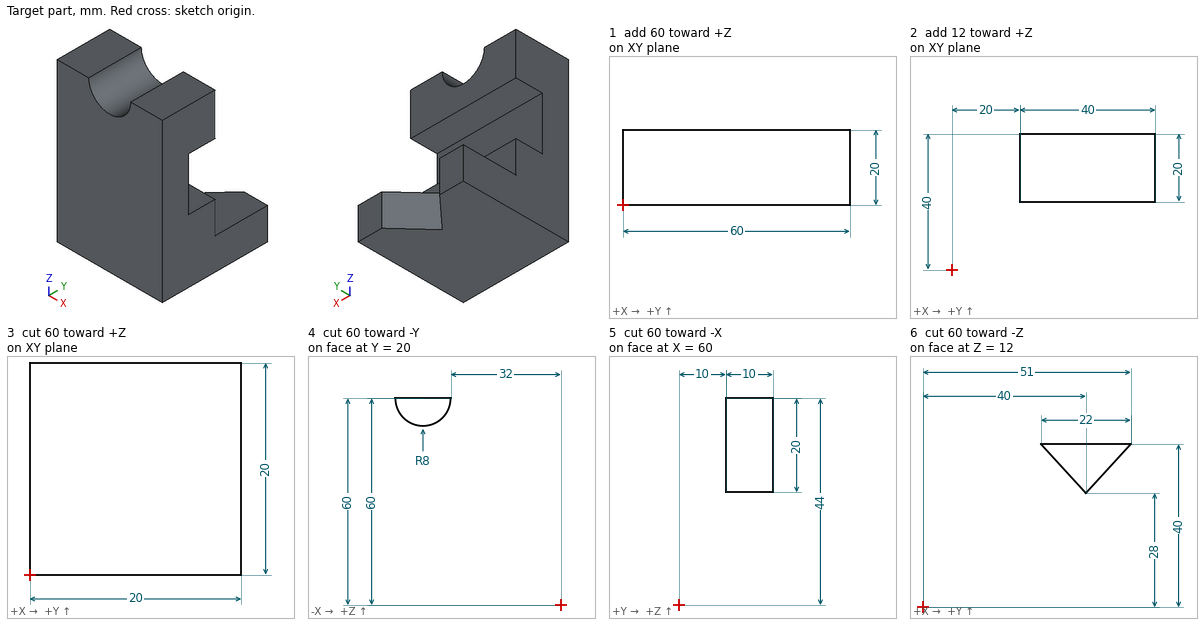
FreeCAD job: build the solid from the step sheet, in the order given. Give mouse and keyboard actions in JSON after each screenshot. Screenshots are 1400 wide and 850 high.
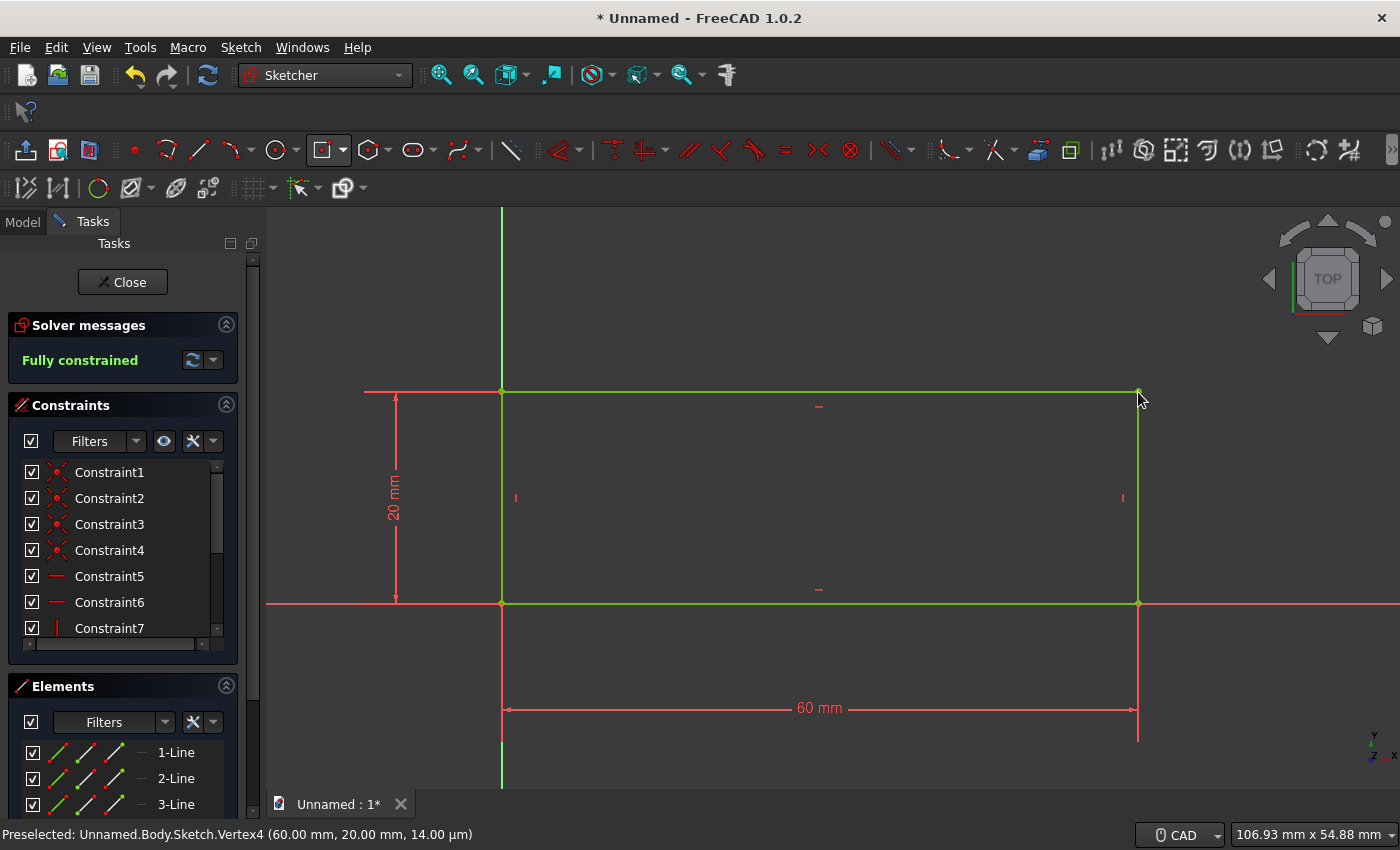
{"action": "left_click", "coordinate": [123, 282]}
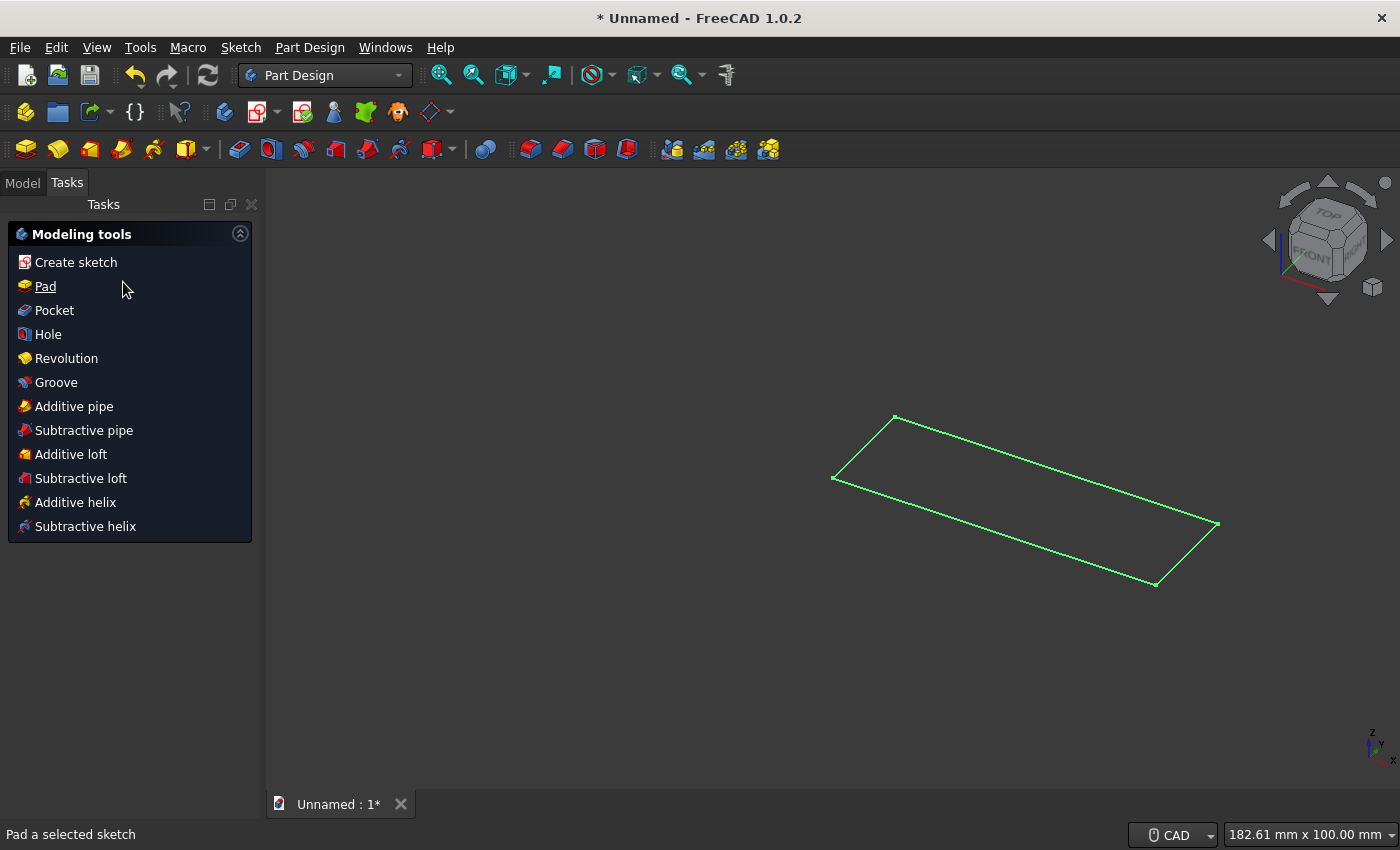
{"action": "left_click", "coordinate": [26, 150]}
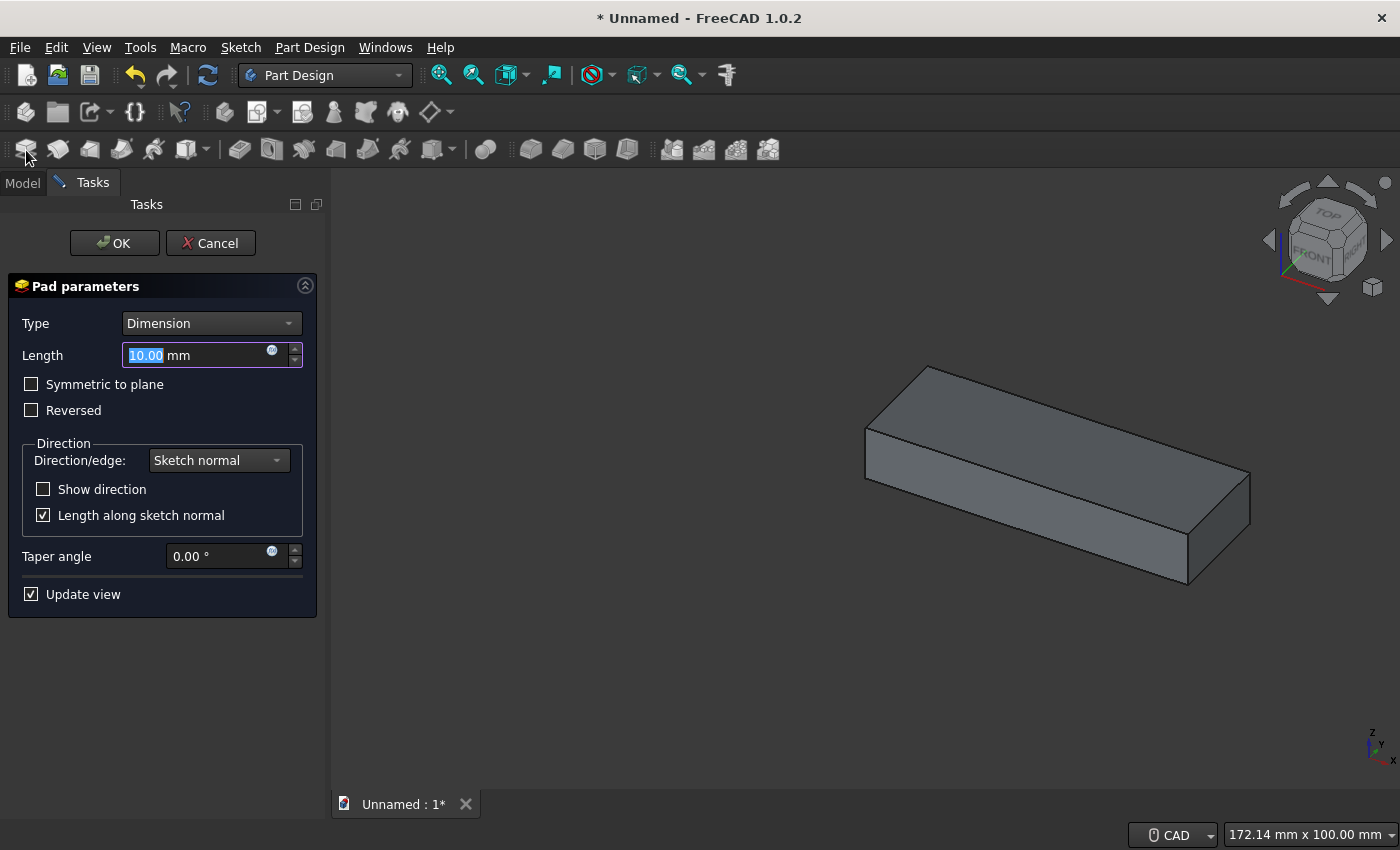
{"action": "type", "text": "60"}
{"action": "key", "text": "Tab"}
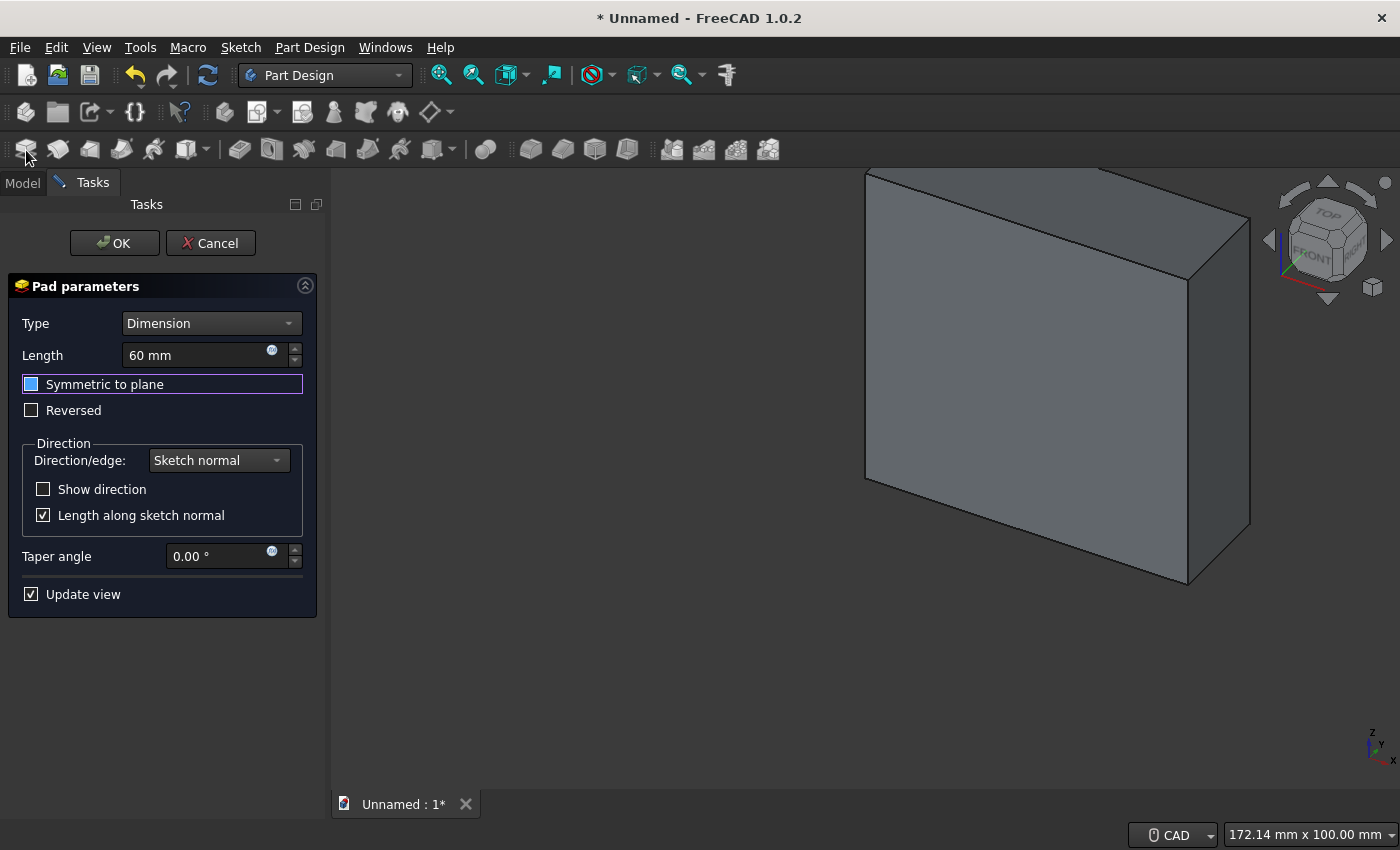
{"action": "left_click", "coordinate": [115, 243]}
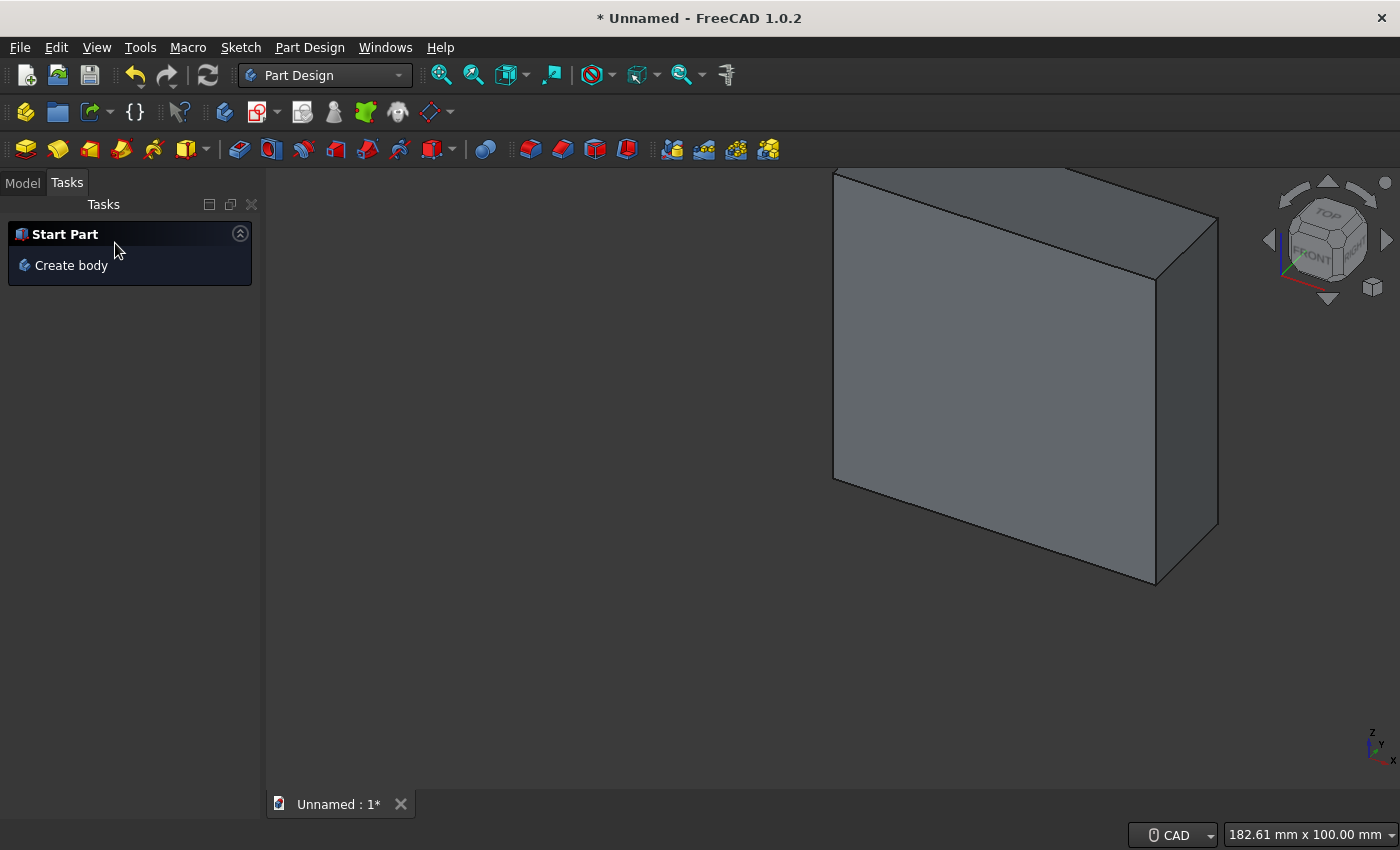
{"action": "left_click", "coordinate": [442, 76]}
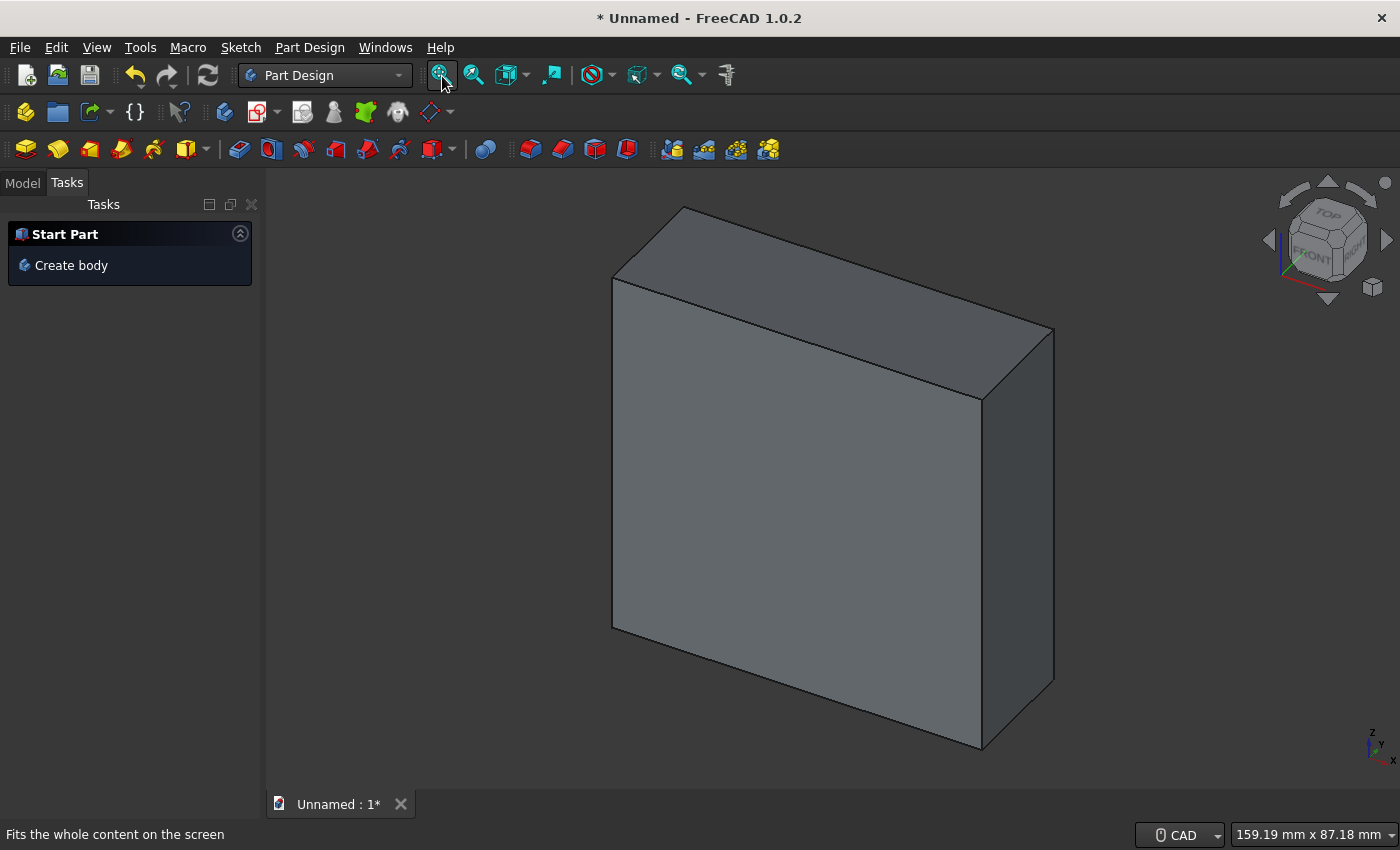
{"action": "left_click", "coordinate": [258, 112]}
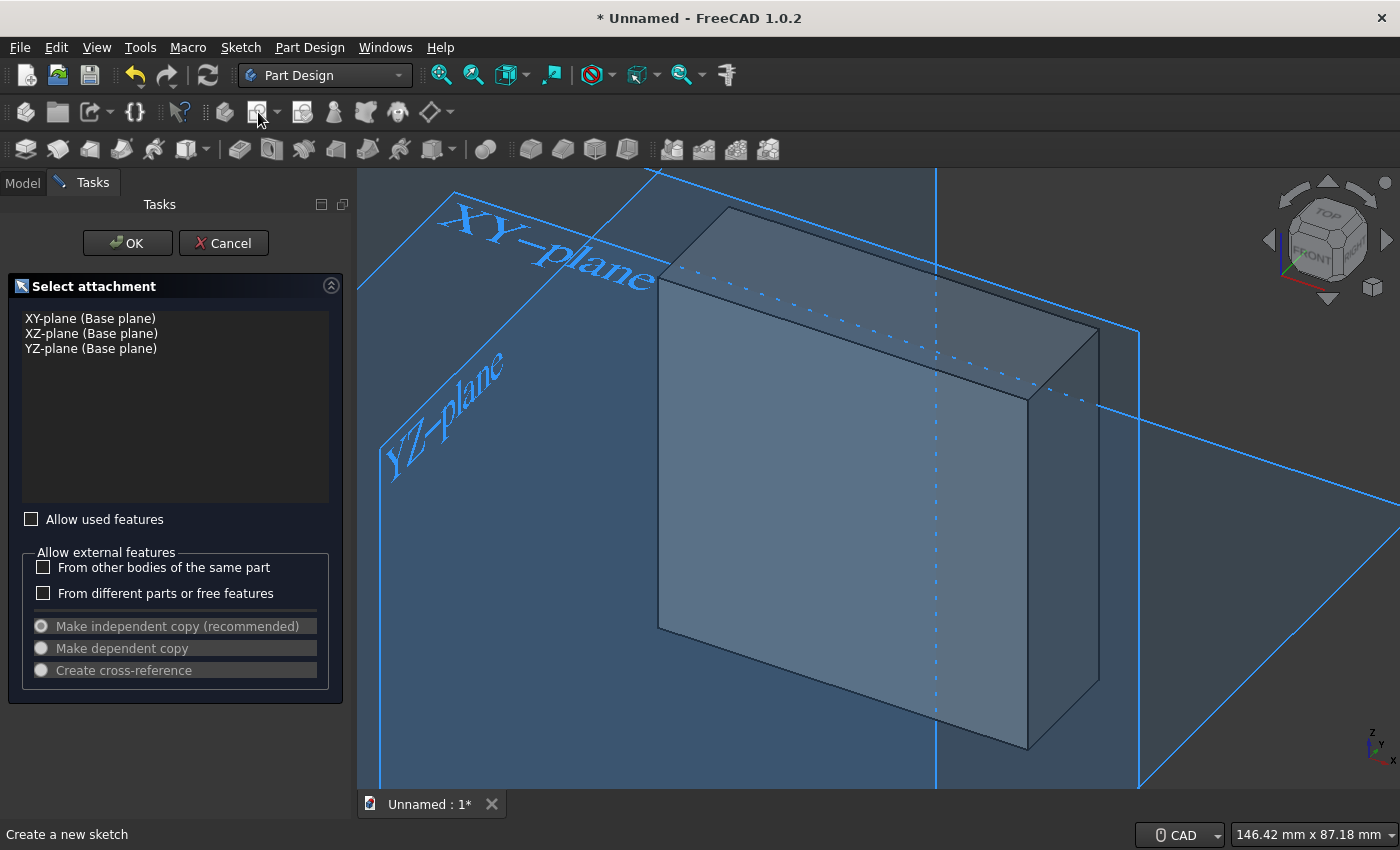
{"action": "left_click", "coordinate": [82, 318]}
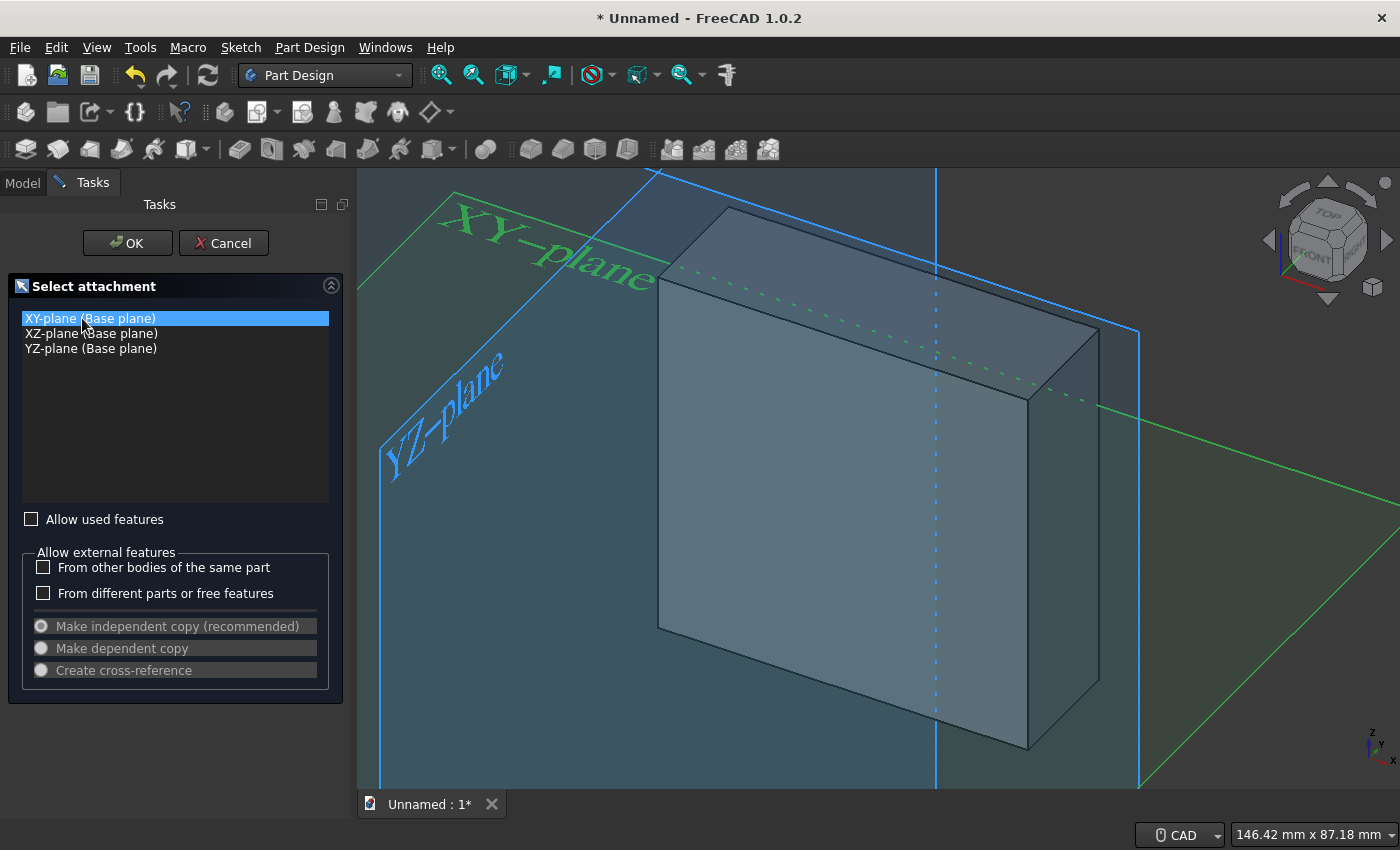
{"action": "left_click", "coordinate": [128, 243]}